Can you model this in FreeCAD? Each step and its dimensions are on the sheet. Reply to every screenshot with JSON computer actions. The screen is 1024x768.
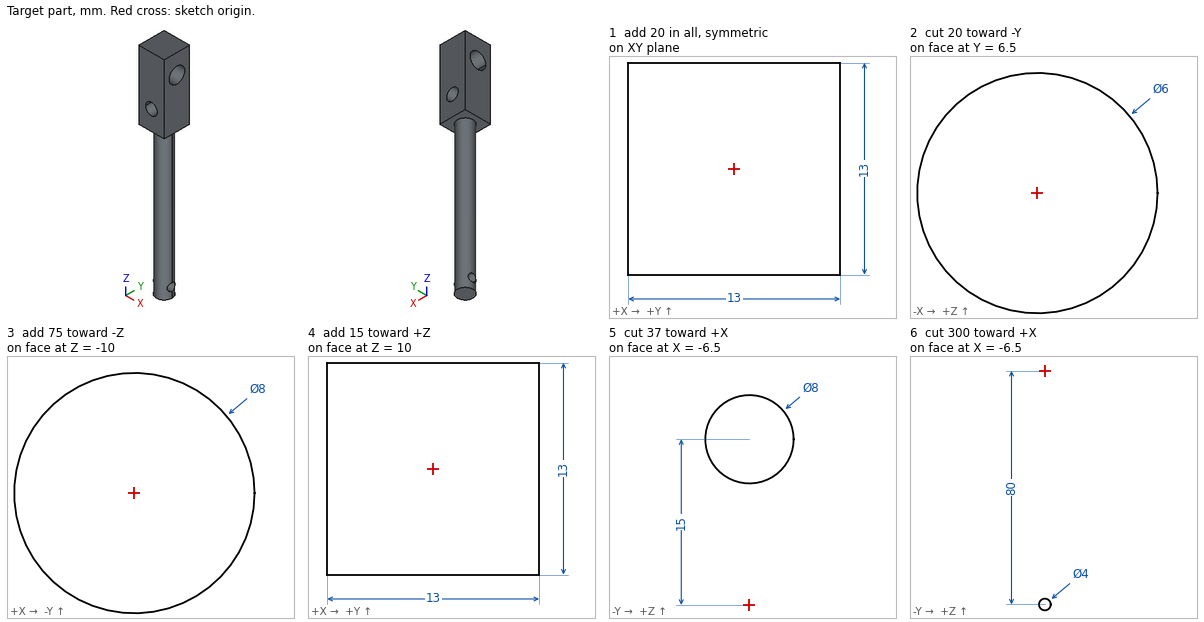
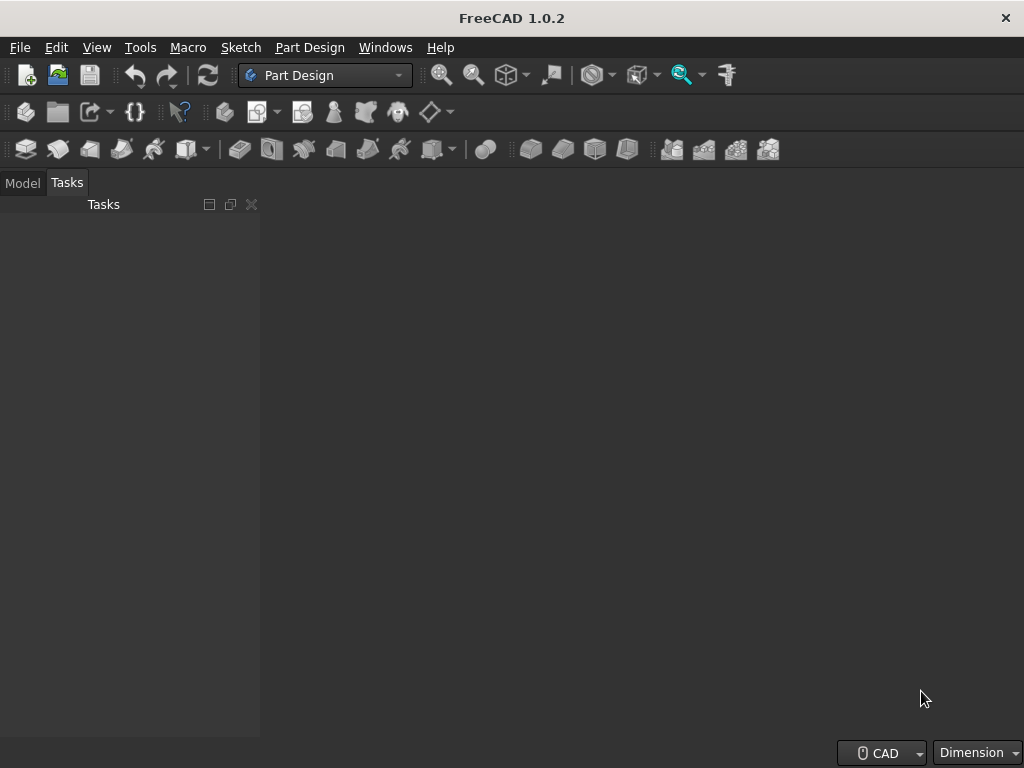
{"action": "left_click", "coordinate": [26, 76]}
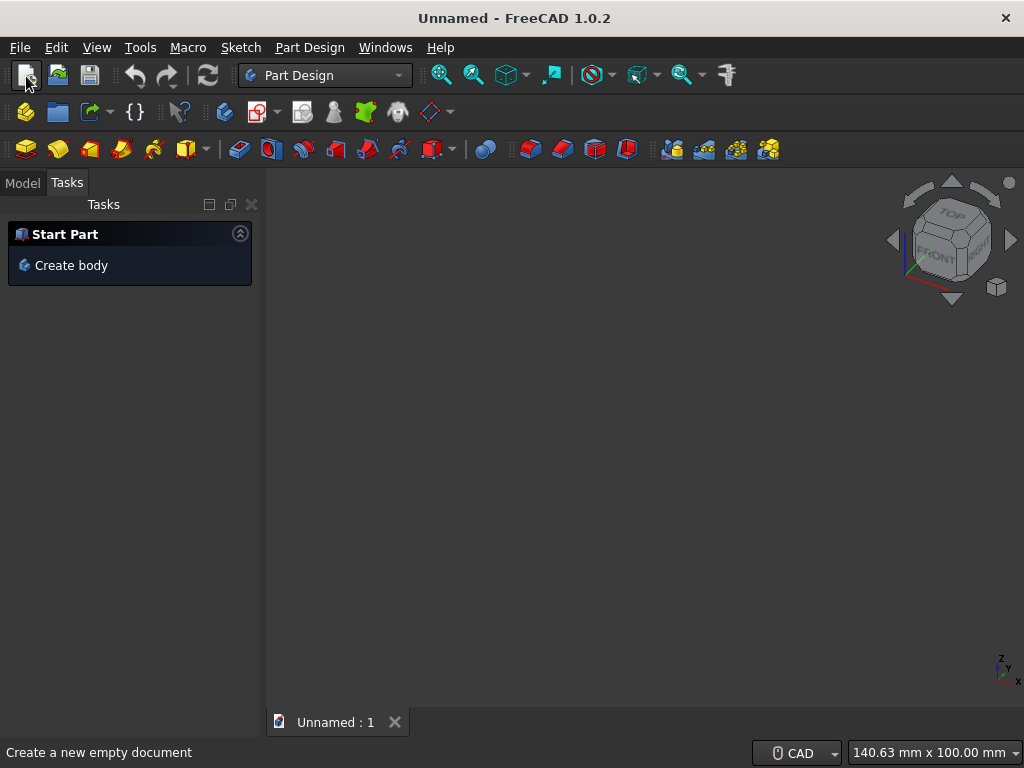
{"action": "left_click", "coordinate": [258, 112]}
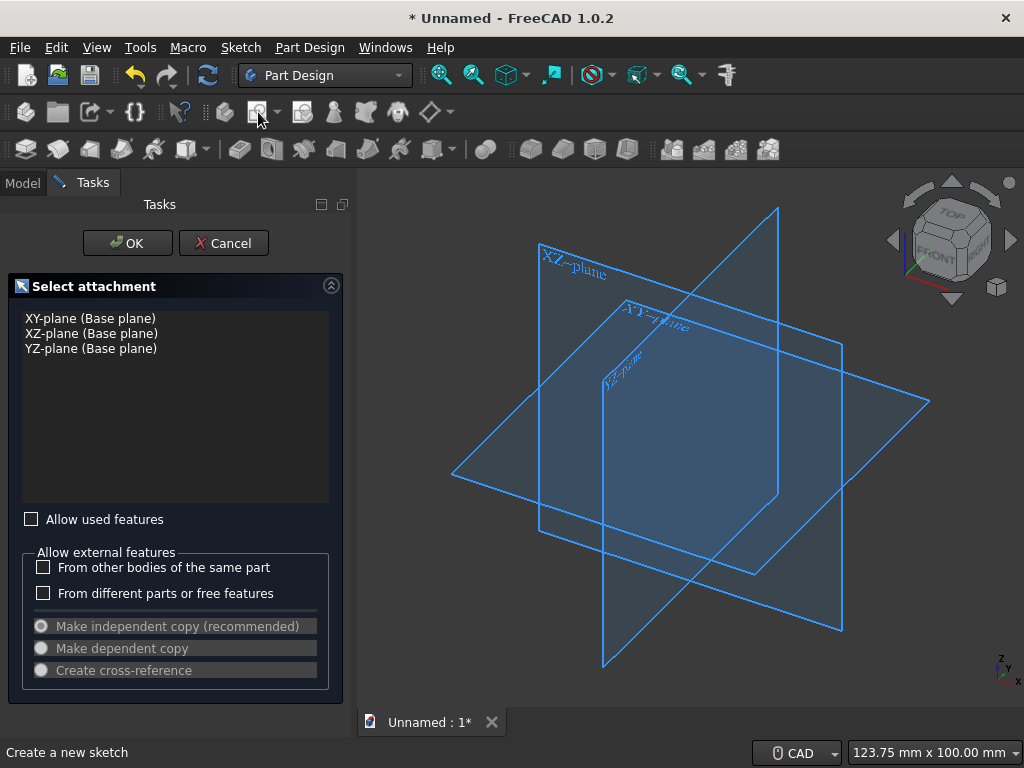
{"action": "left_click", "coordinate": [82, 318]}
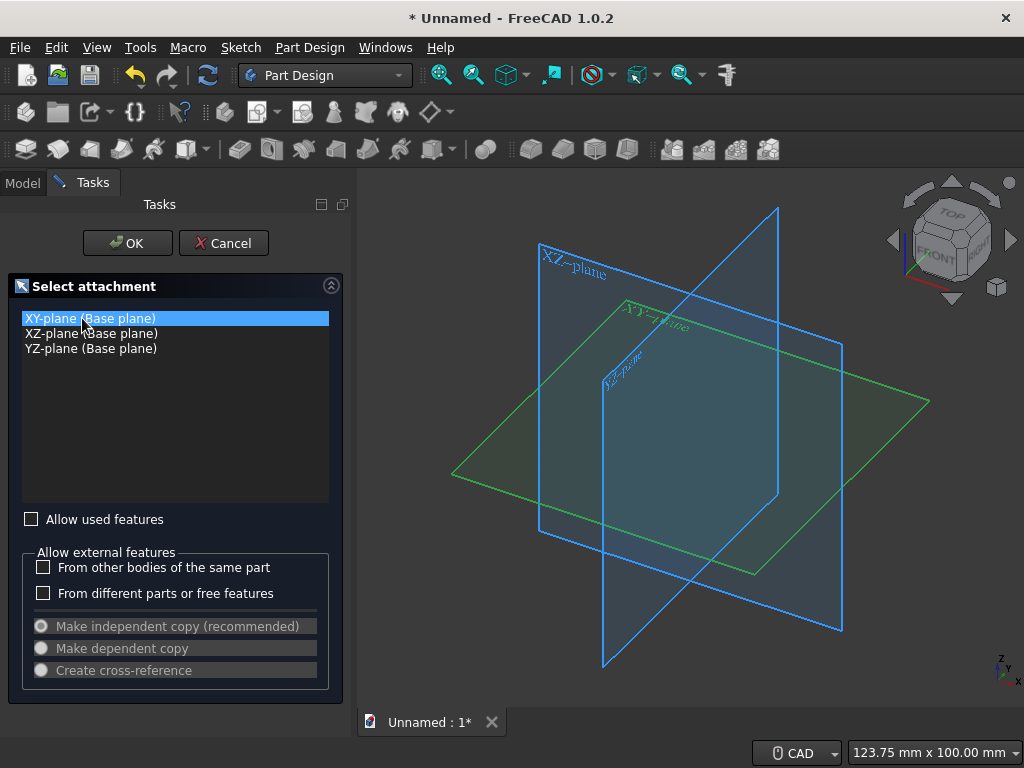
{"action": "left_click", "coordinate": [128, 243]}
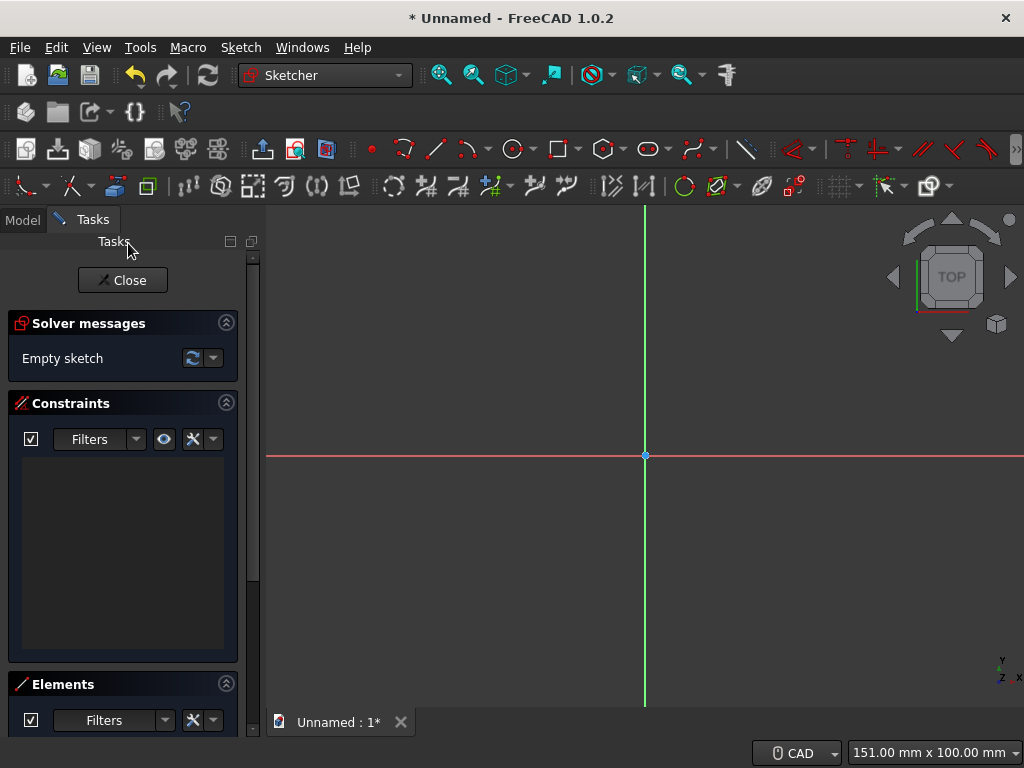
{"action": "scroll", "coordinate": [662, 456], "scroll_direction": "up", "scroll_amount": 8}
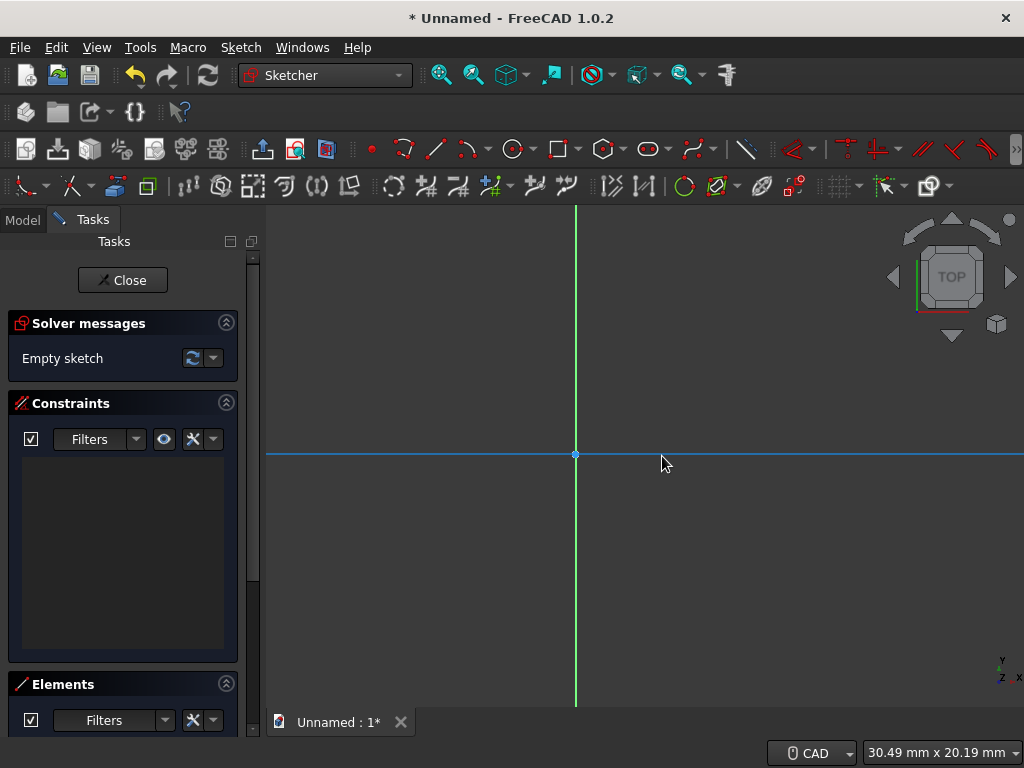
{"action": "left_click", "coordinate": [580, 150]}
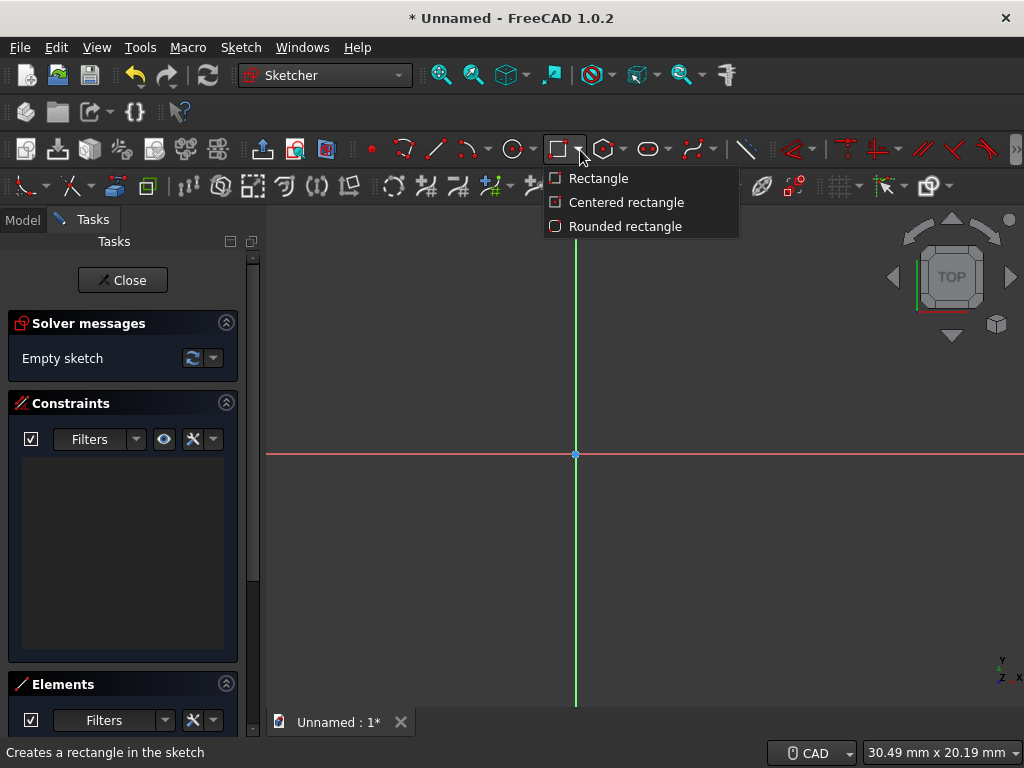
{"action": "left_click", "coordinate": [642, 202]}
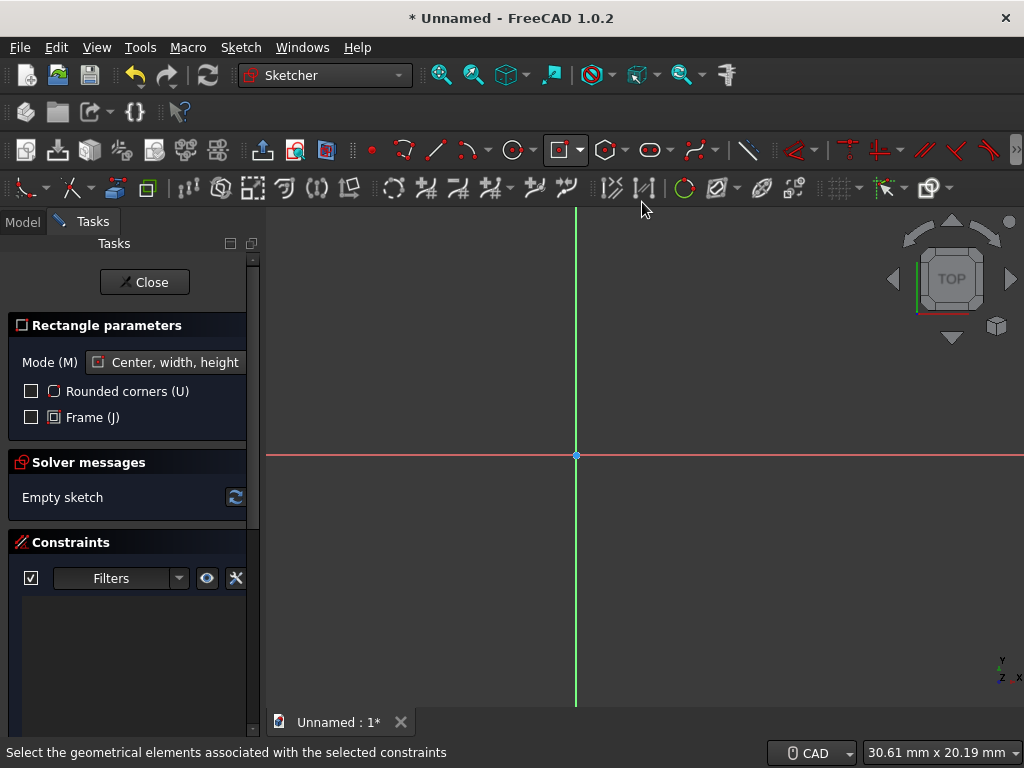
{"action": "left_click", "coordinate": [576, 455]}
{"action": "mouse_move", "coordinate": [737, 294]}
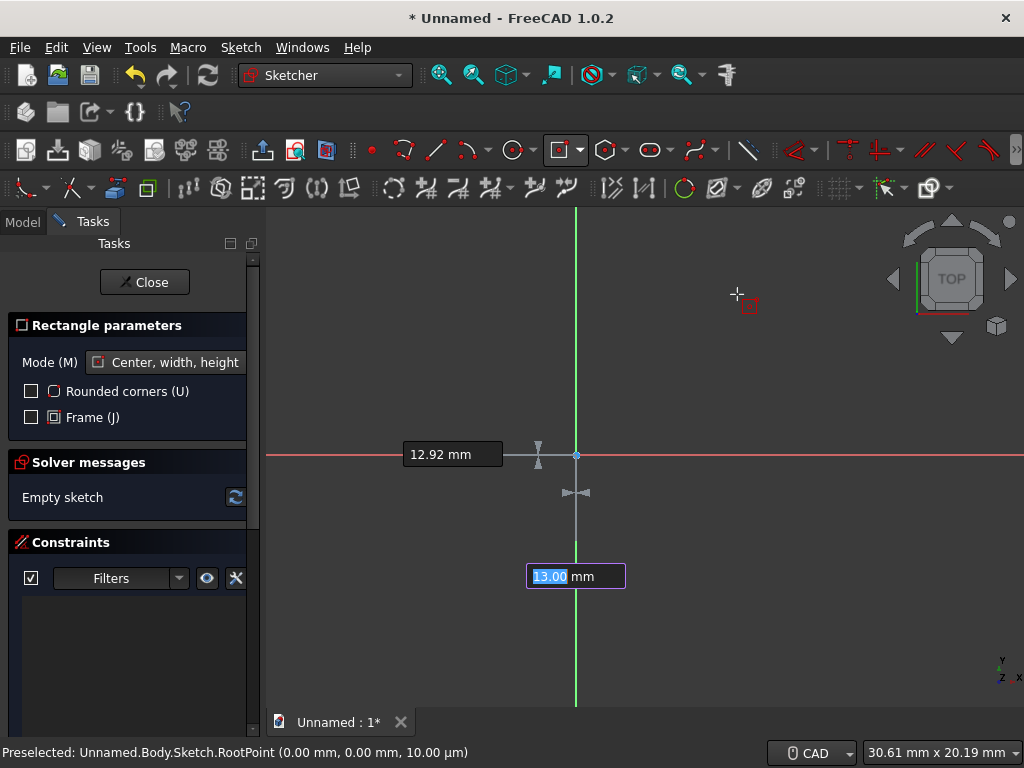
{"action": "type", "text": "13"}
{"action": "key", "text": "Tab"}
{"action": "type", "text": "13"}
{"action": "key", "text": "Return"}
{"action": "key", "text": "Escape"}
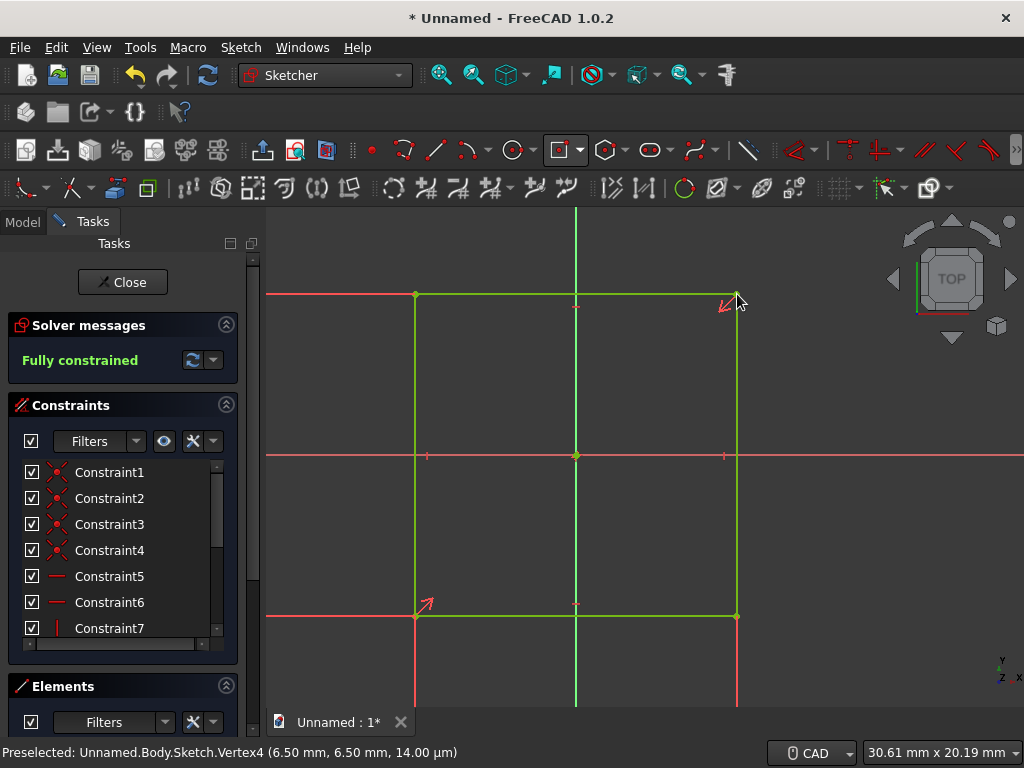
{"action": "left_click", "coordinate": [123, 282]}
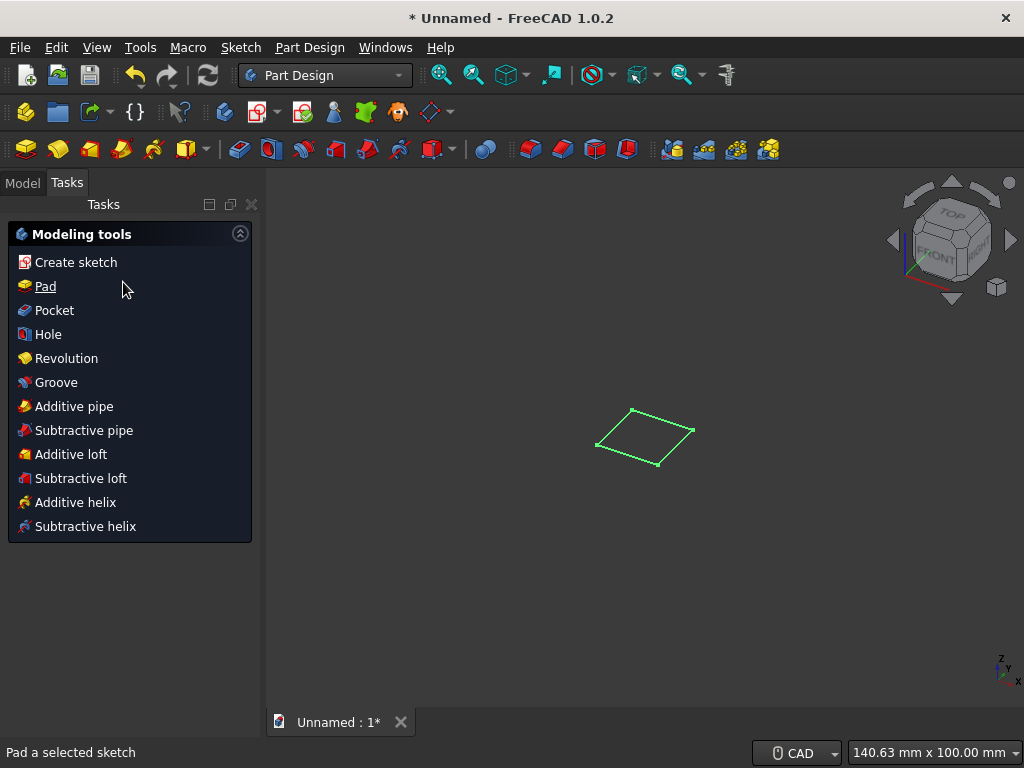
{"action": "left_click", "coordinate": [26, 150]}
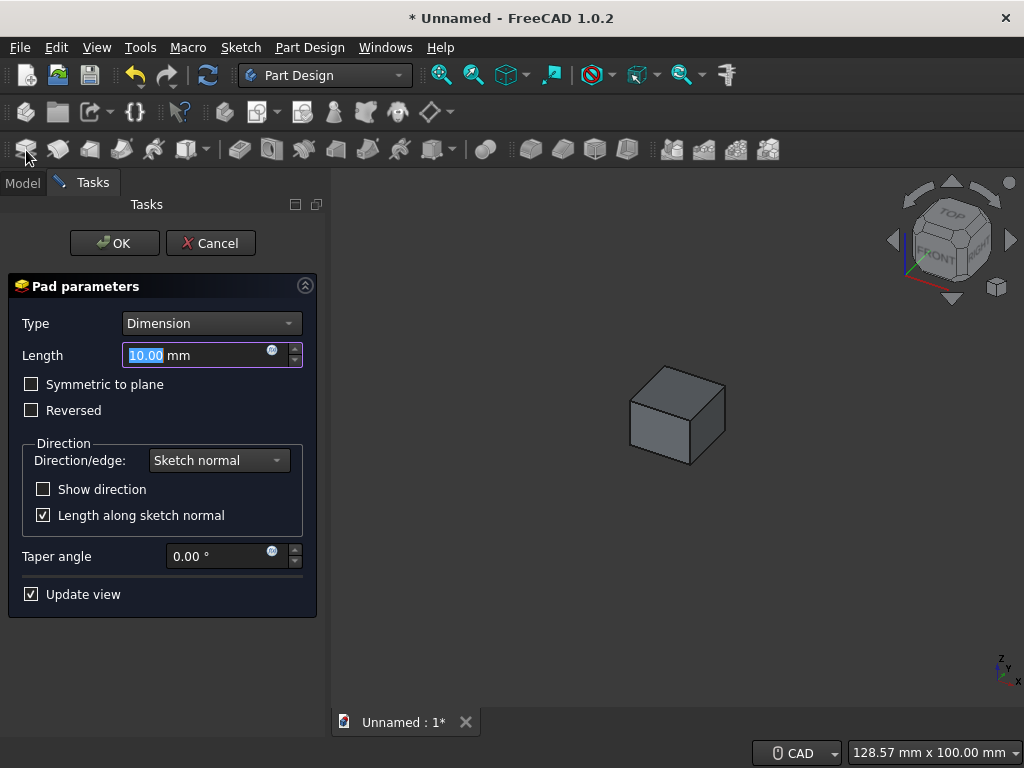
{"action": "type", "text": "20"}
{"action": "key", "text": "Tab"}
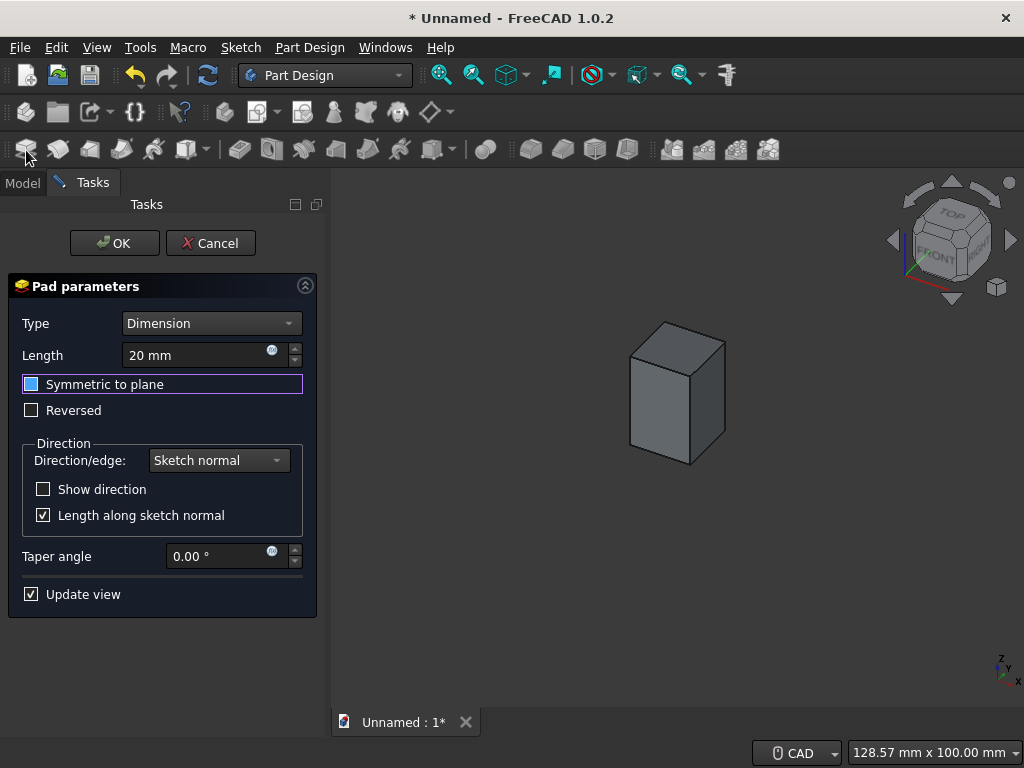
{"action": "left_click", "coordinate": [30, 384]}